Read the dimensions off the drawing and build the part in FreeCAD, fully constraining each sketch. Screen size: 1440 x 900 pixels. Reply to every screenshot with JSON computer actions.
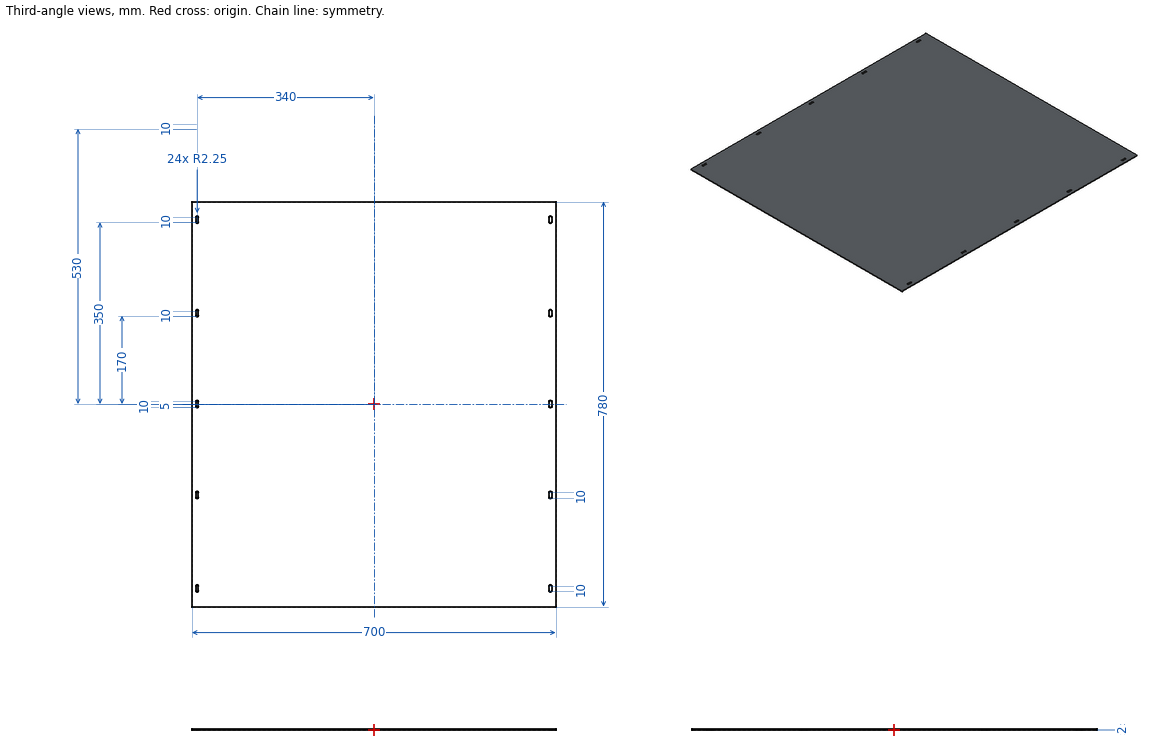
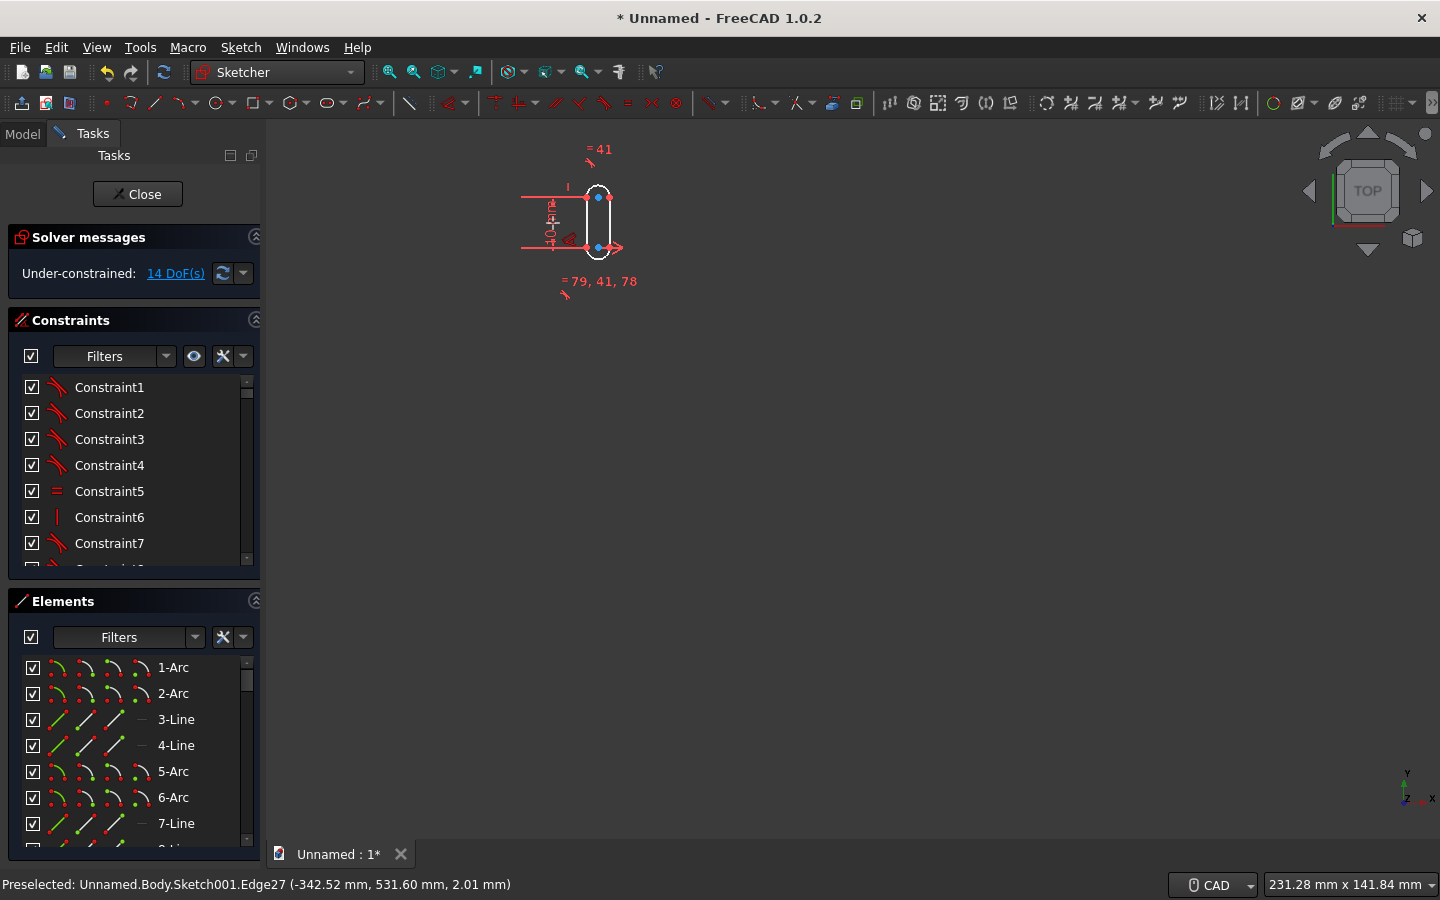
{"action": "scroll", "coordinate": [593, 230], "scroll_direction": "down", "scroll_amount": 11}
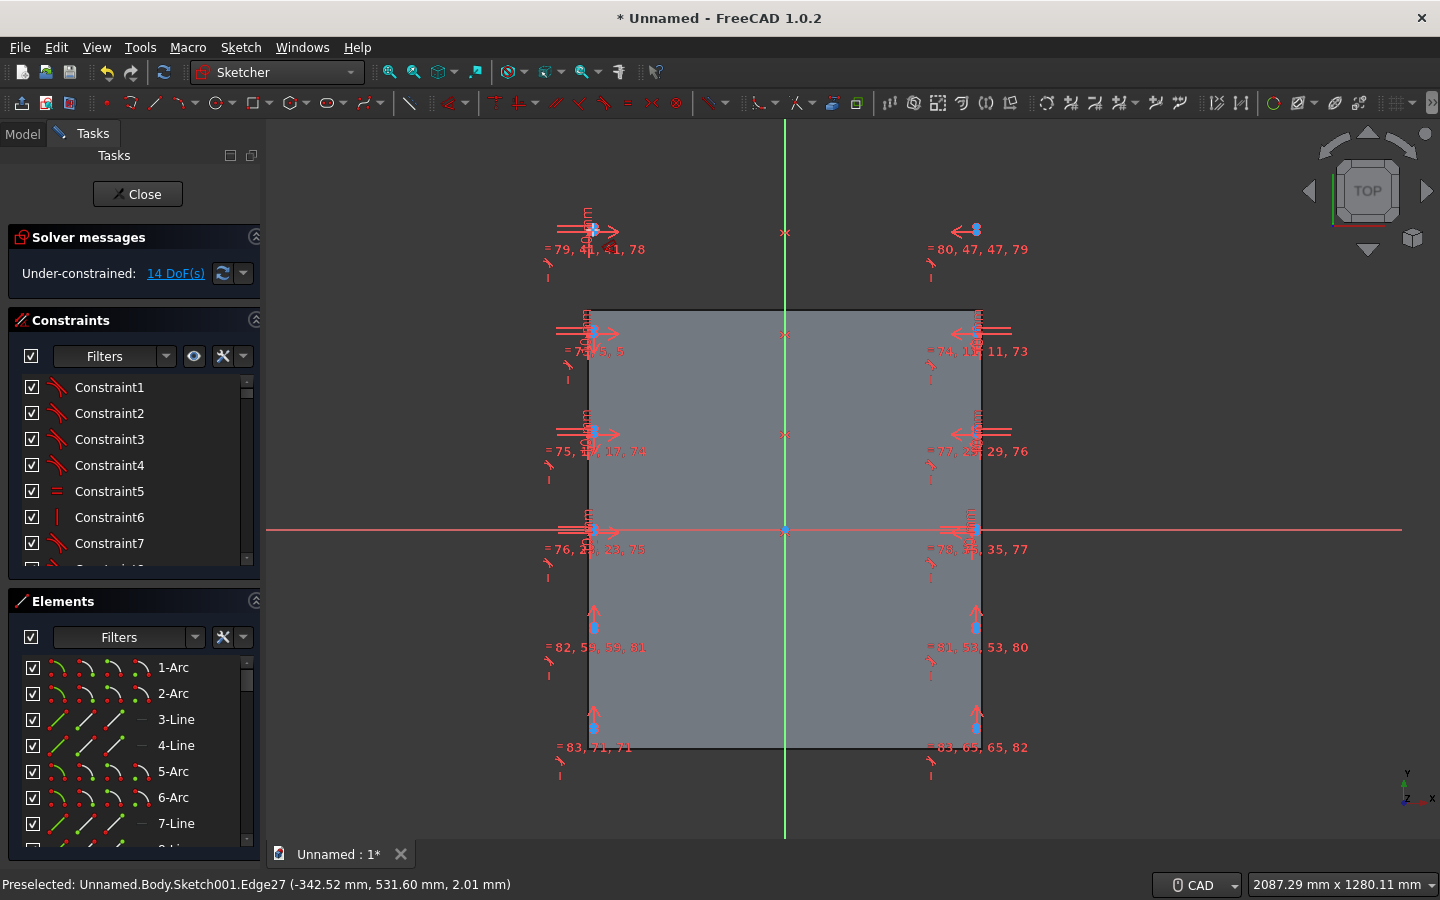
{"action": "scroll", "coordinate": [975, 230], "scroll_direction": "up", "scroll_amount": 11}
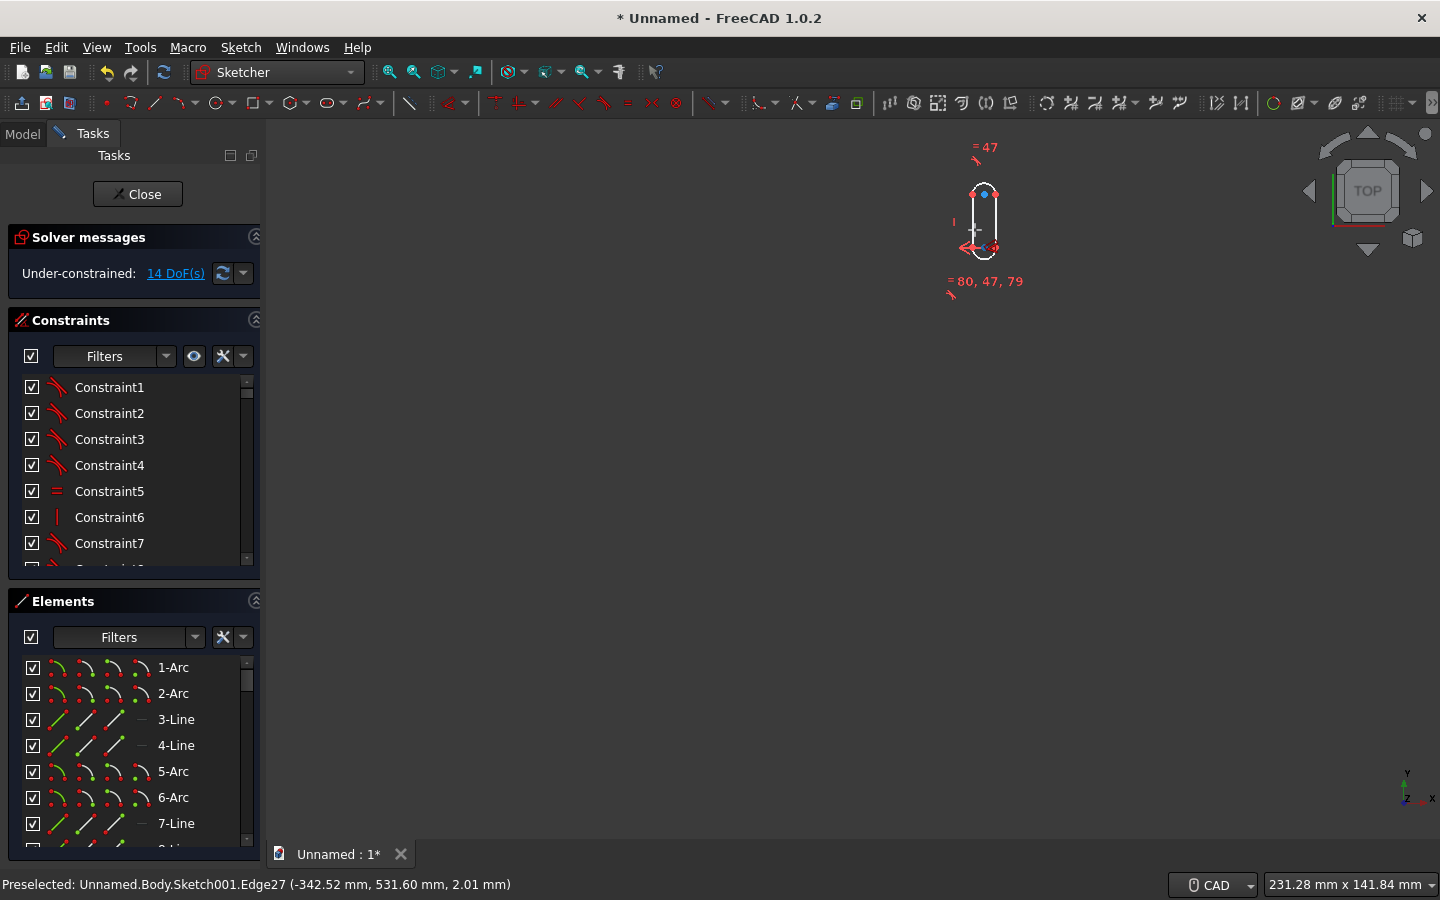
{"action": "left_click", "coordinate": [973, 232]}
{"action": "left_click", "coordinate": [939, 221]}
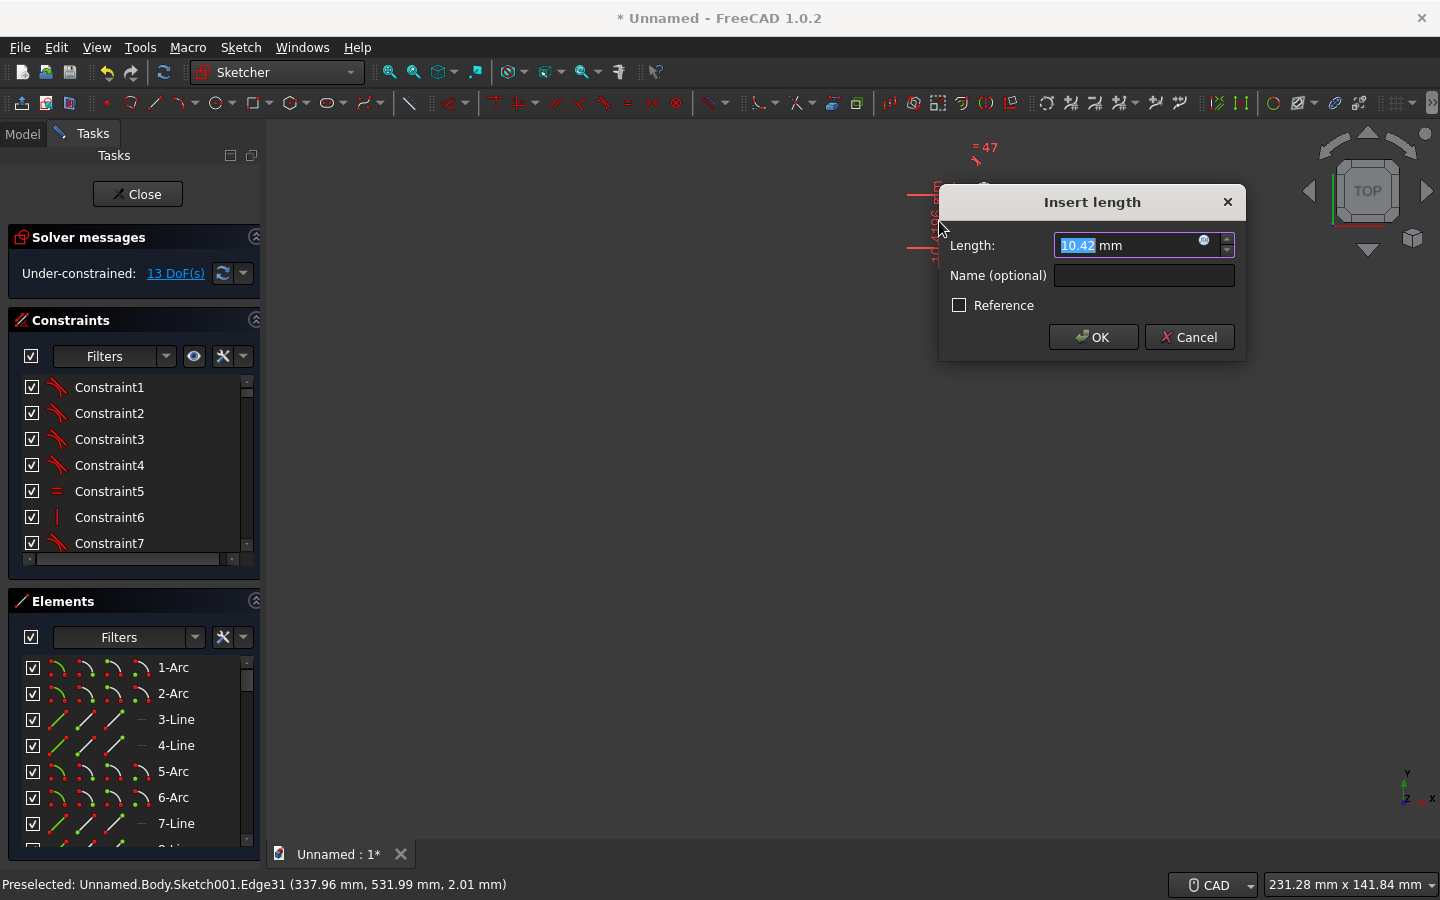
{"action": "type", "text": "10"}
{"action": "key", "text": "Return"}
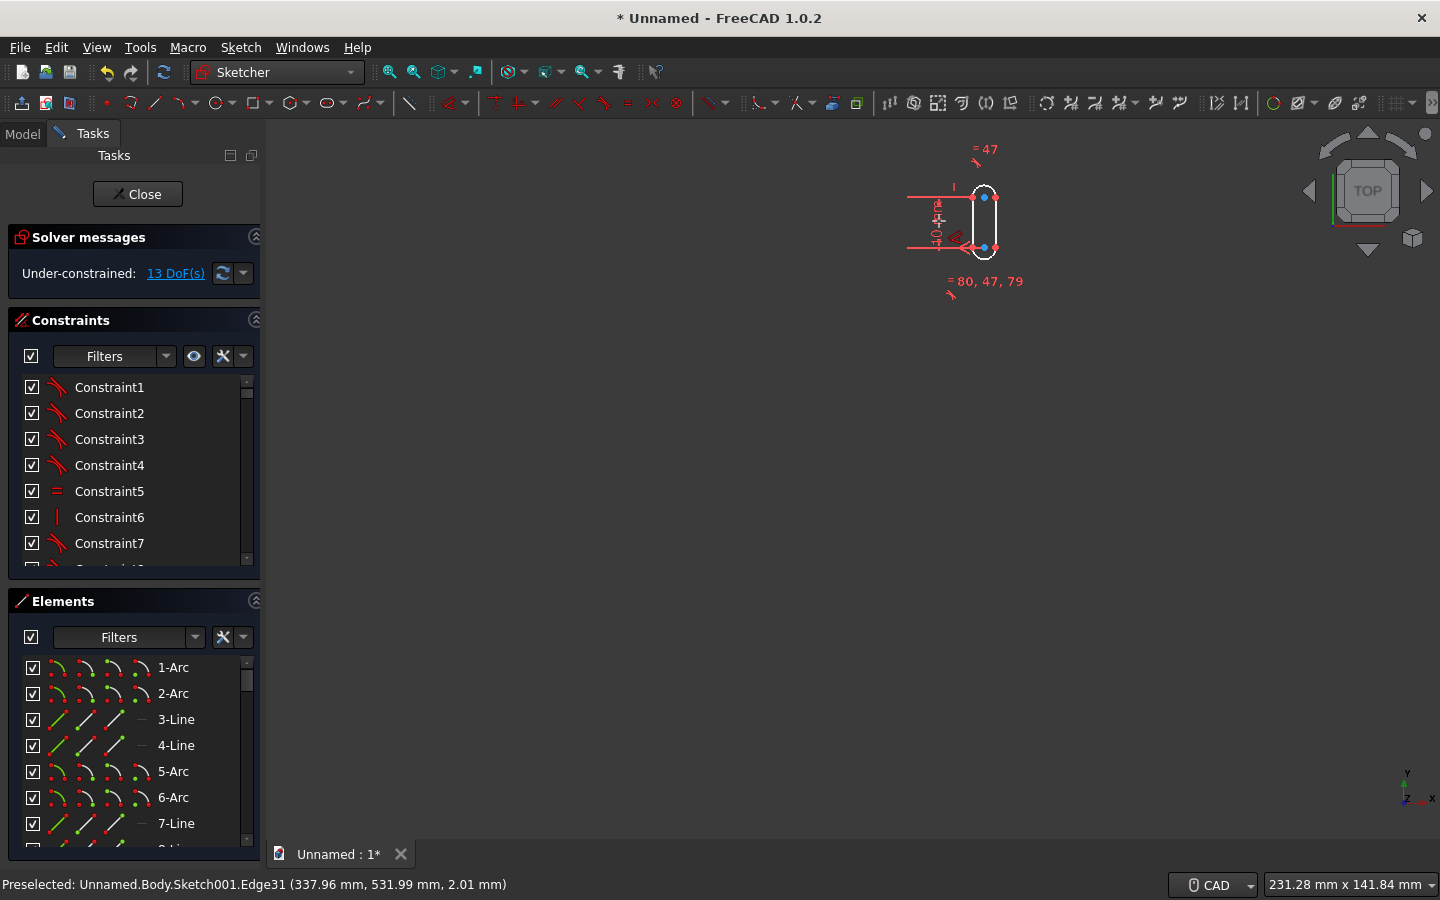
{"action": "scroll", "coordinate": [975, 230], "scroll_direction": "down", "scroll_amount": 11}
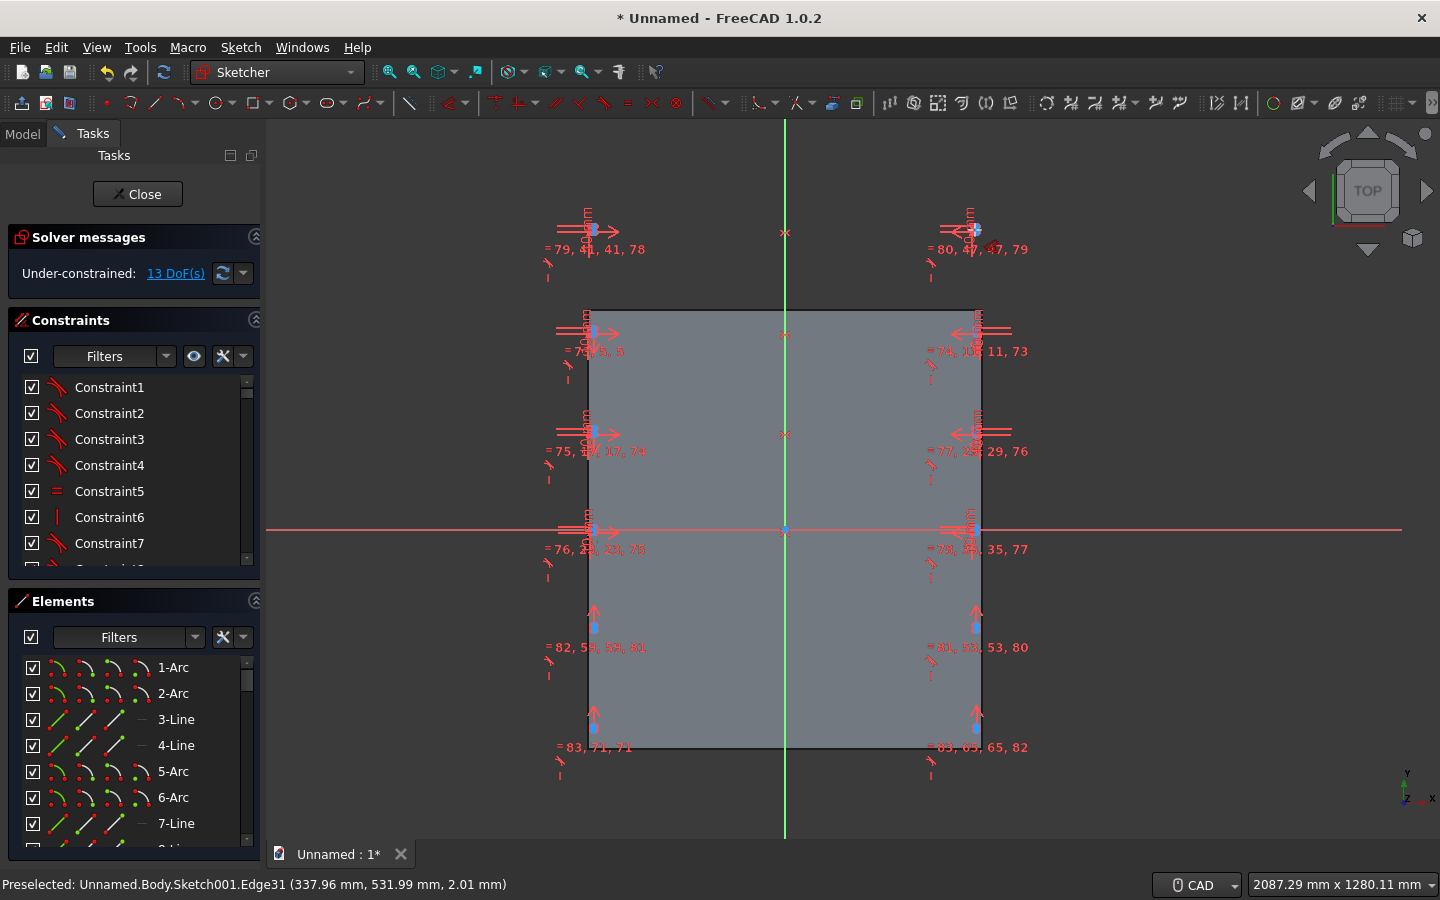
{"action": "scroll", "coordinate": [975, 629], "scroll_direction": "up", "scroll_amount": 12}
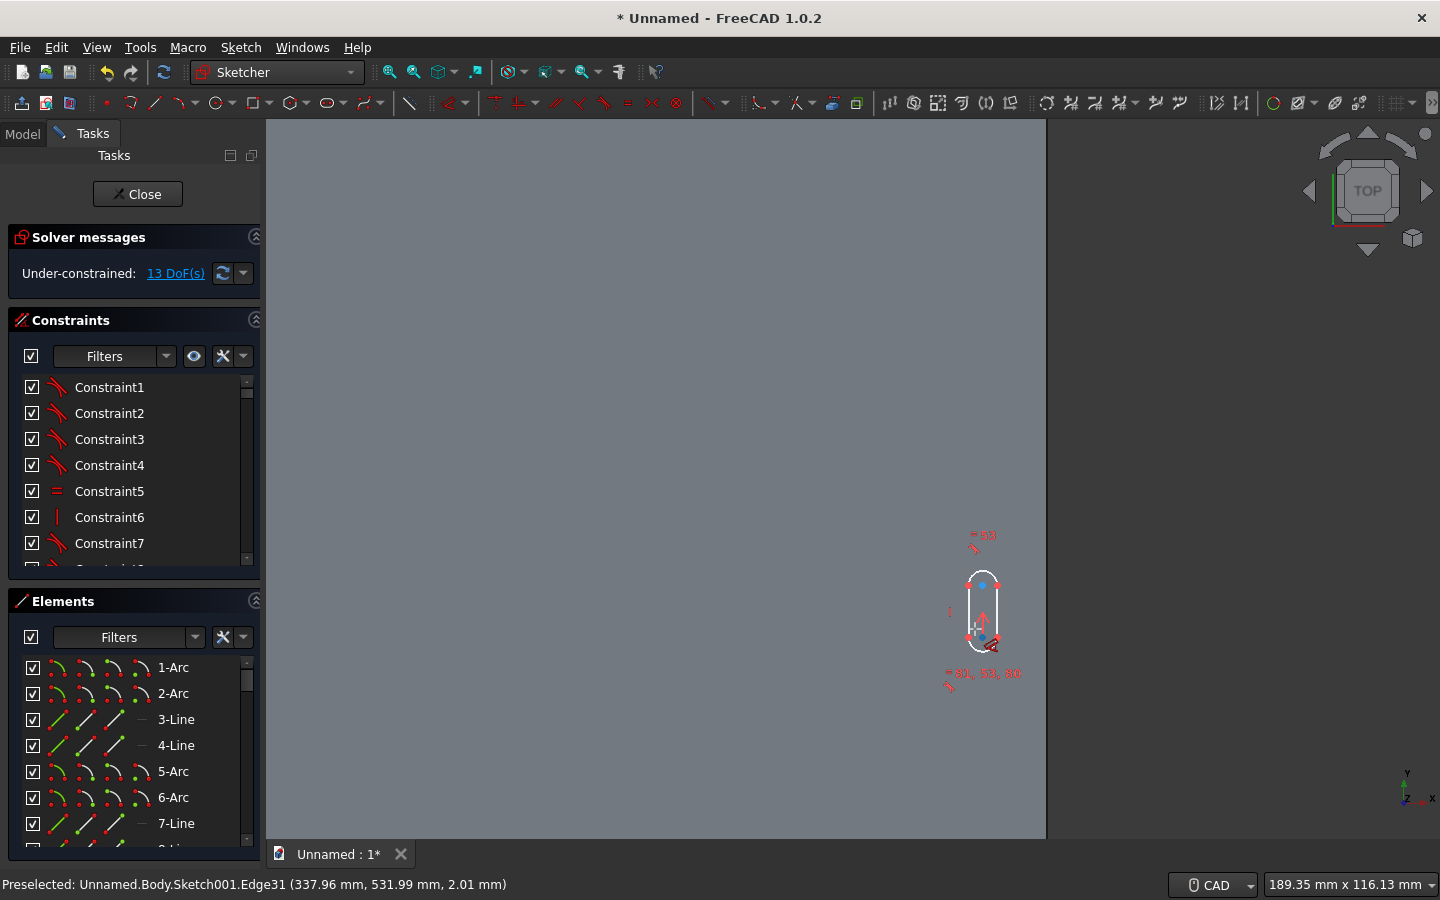
{"action": "left_click", "coordinate": [969, 622]}
{"action": "left_click", "coordinate": [935, 611]}